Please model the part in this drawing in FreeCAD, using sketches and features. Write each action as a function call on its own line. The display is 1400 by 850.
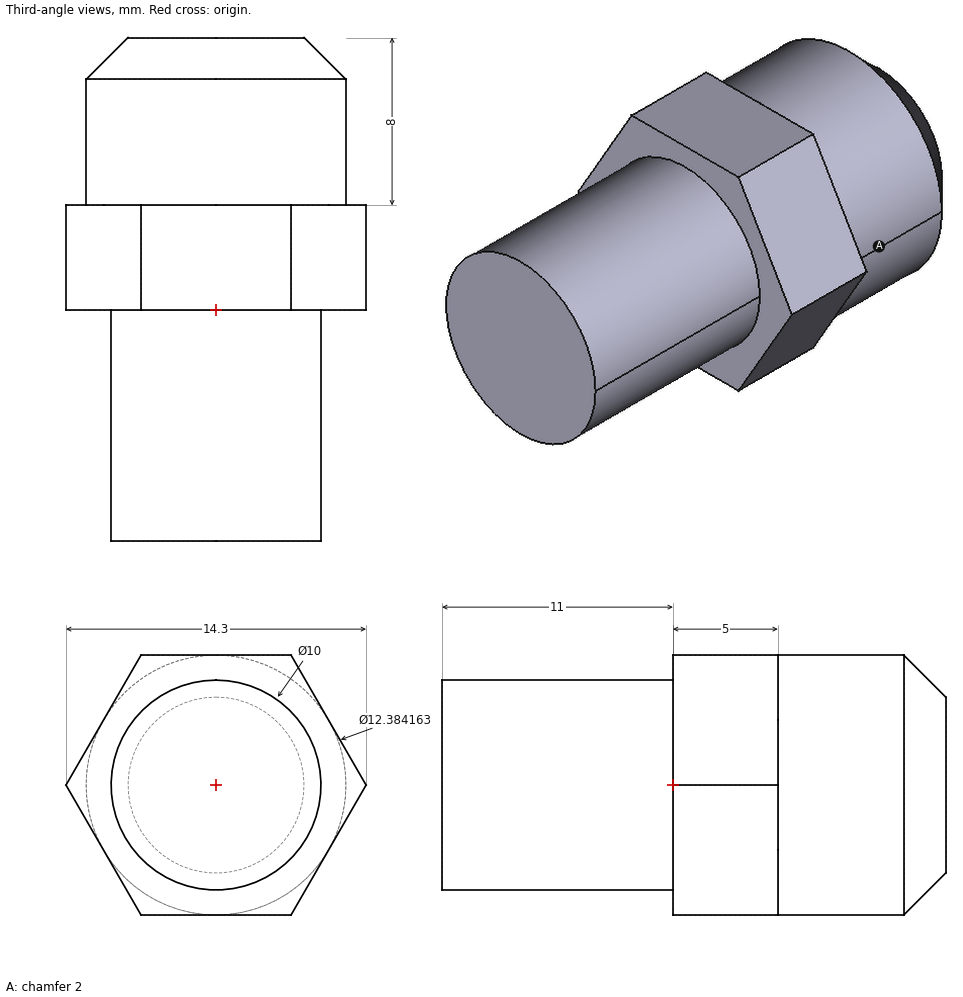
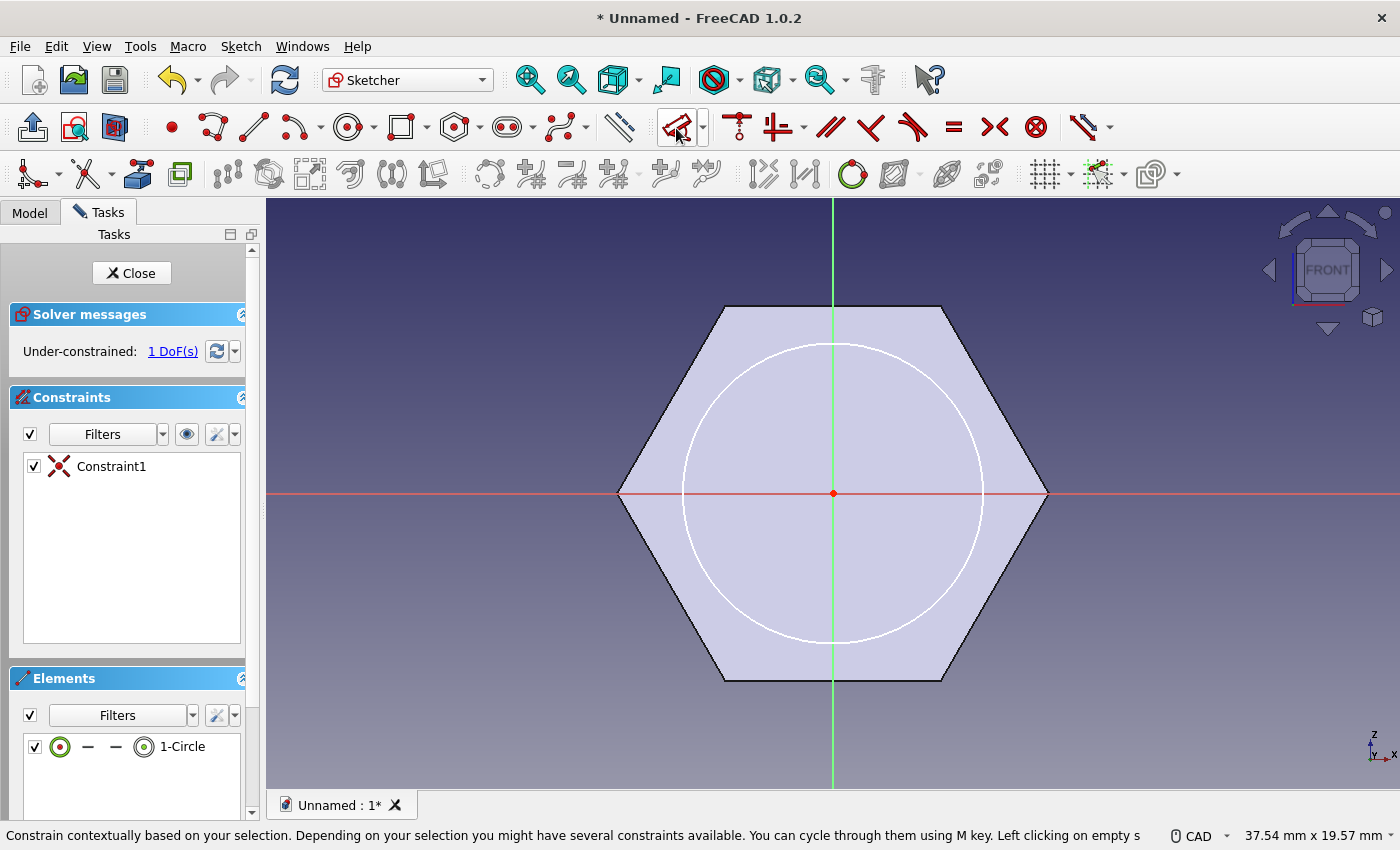
click(939, 387)
click(962, 364)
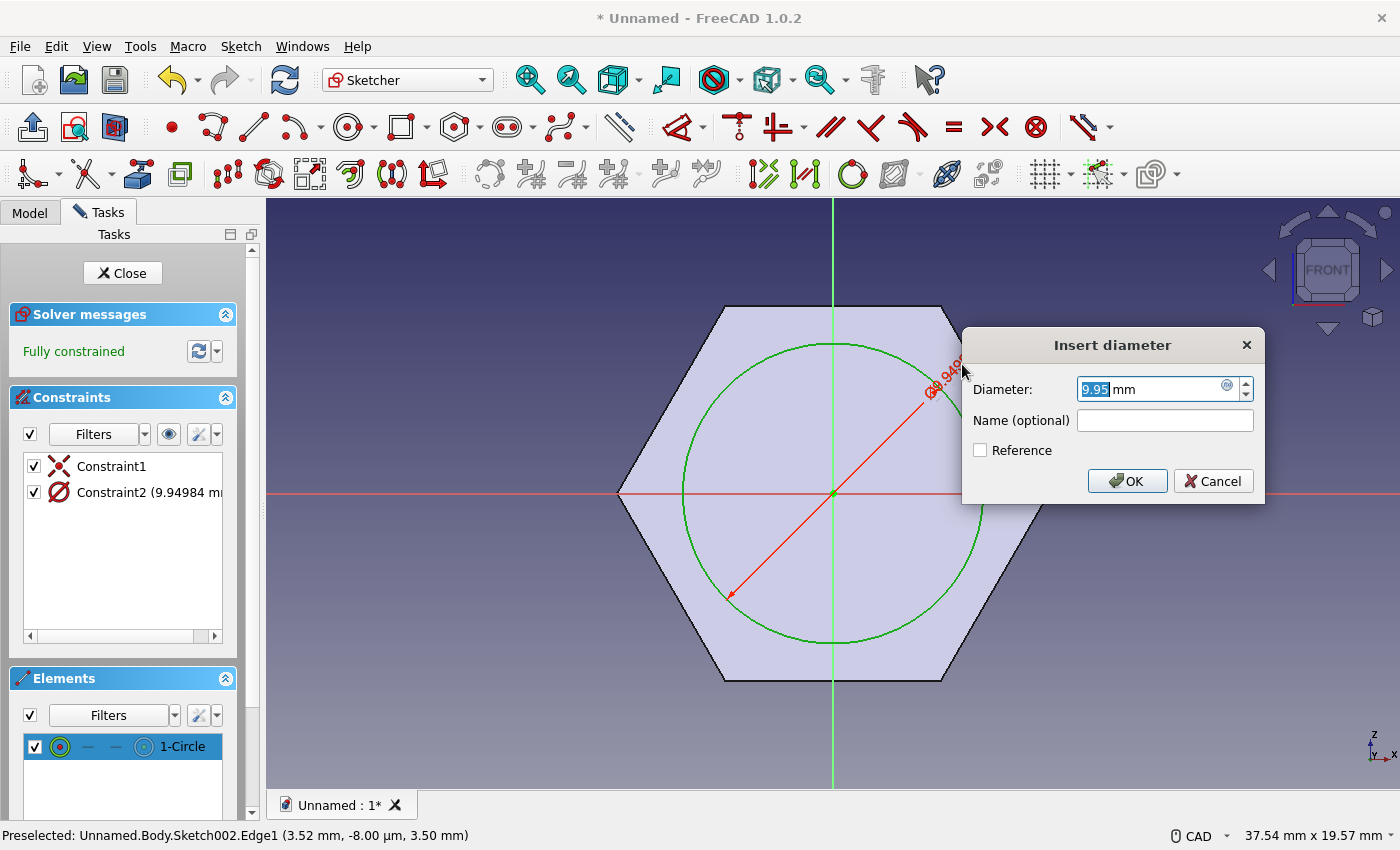
text(10)
key(Return)
key(Escape)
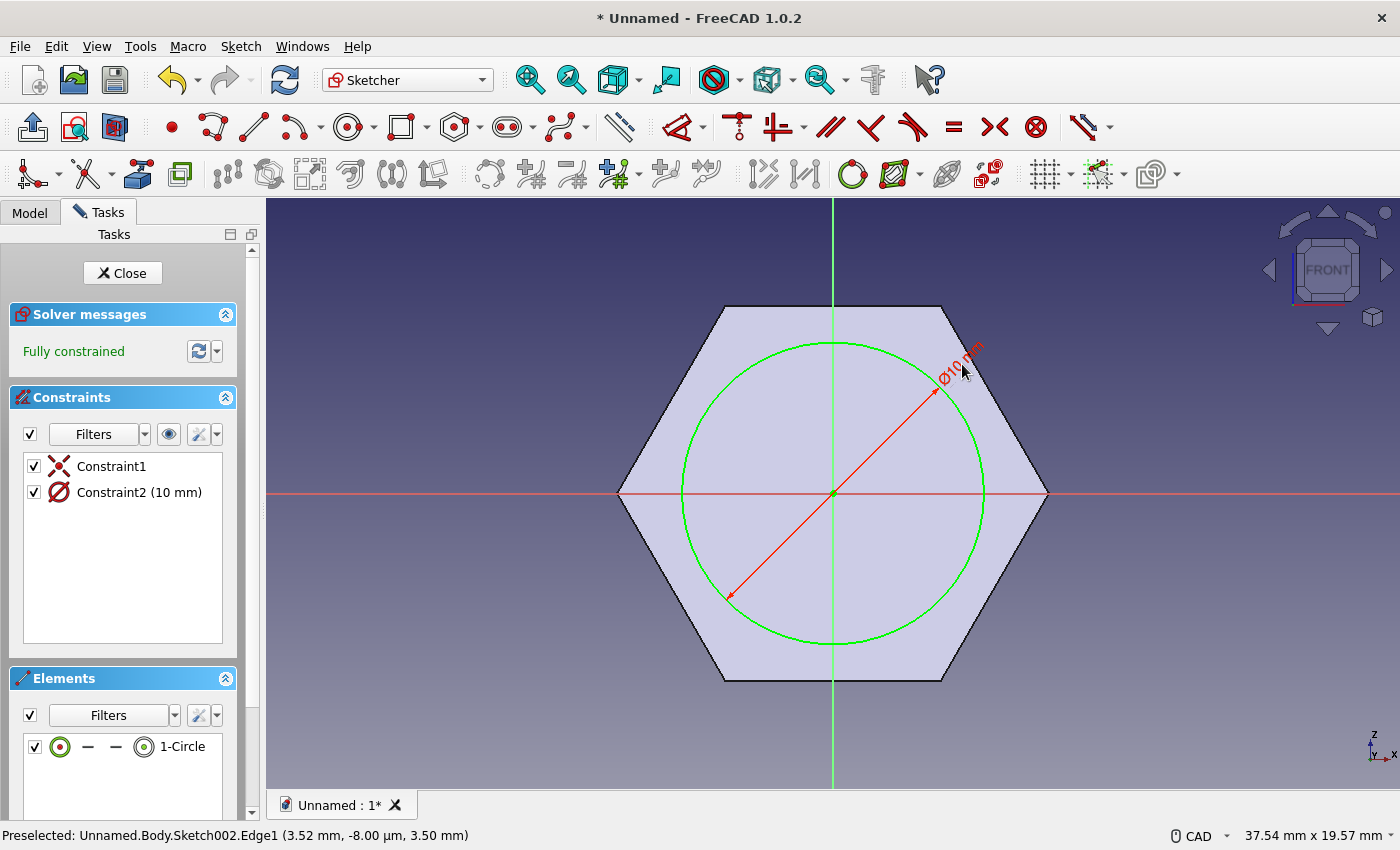
click(123, 273)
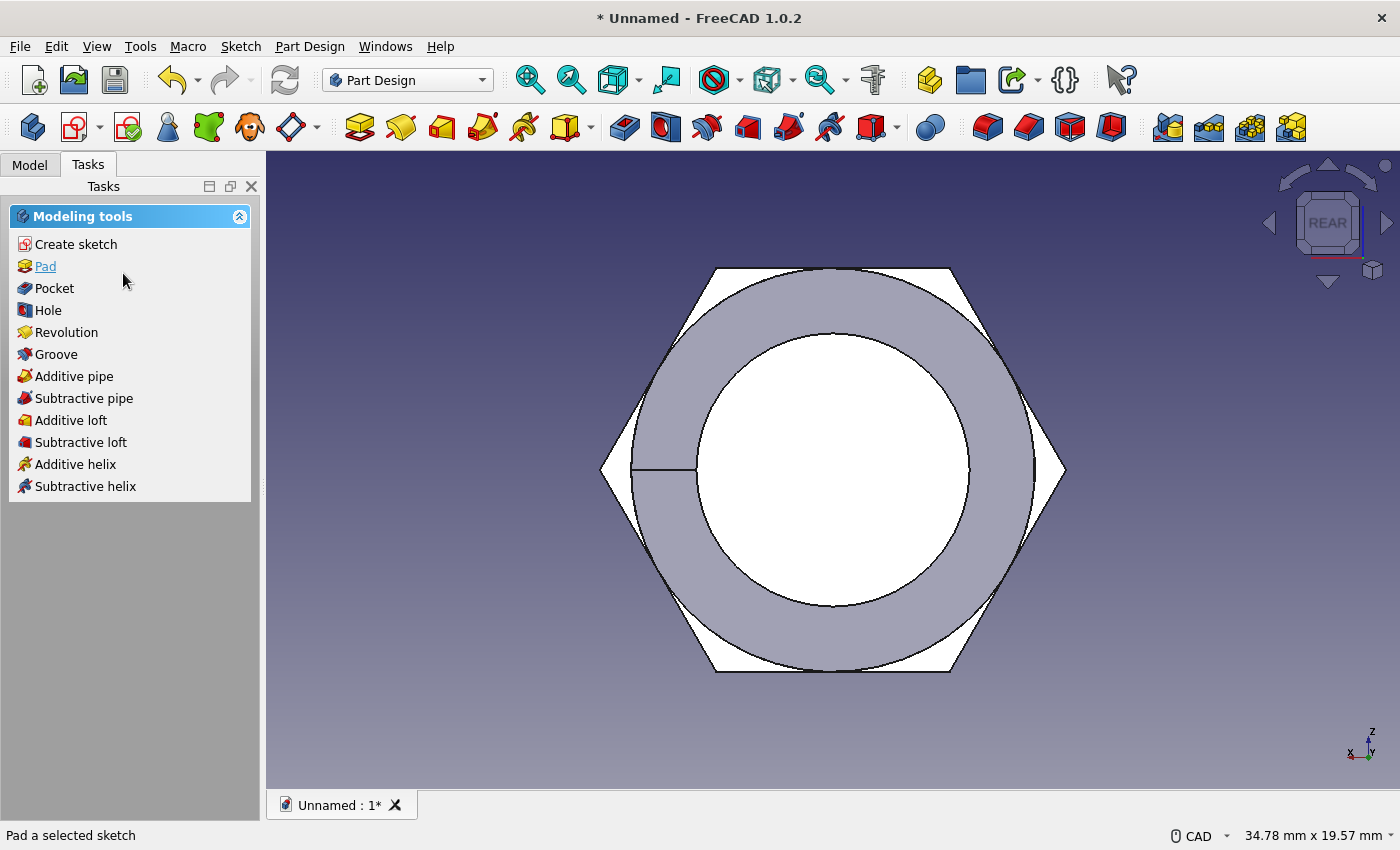
click(360, 128)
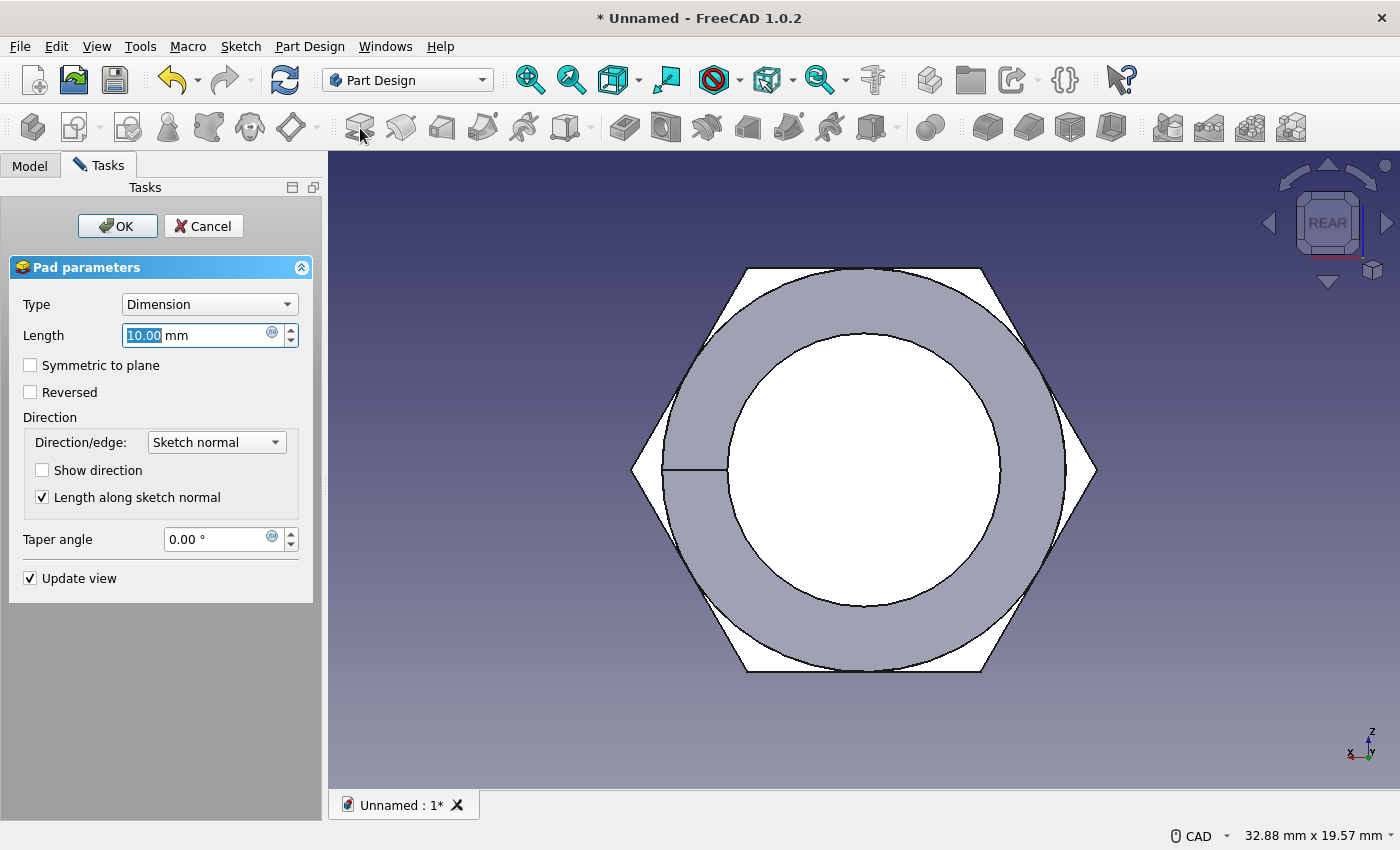
text(11)
key(Tab)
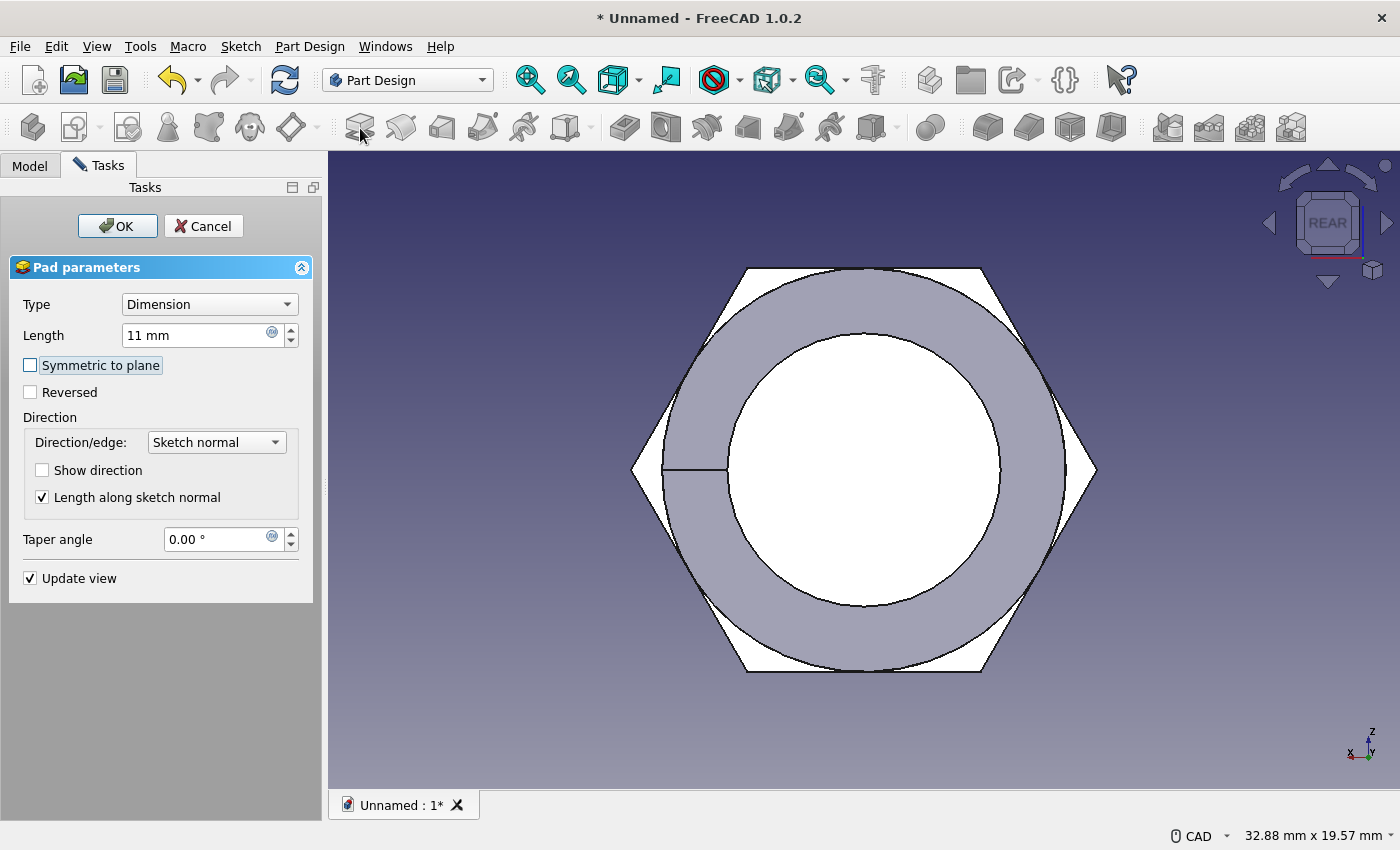
click(118, 226)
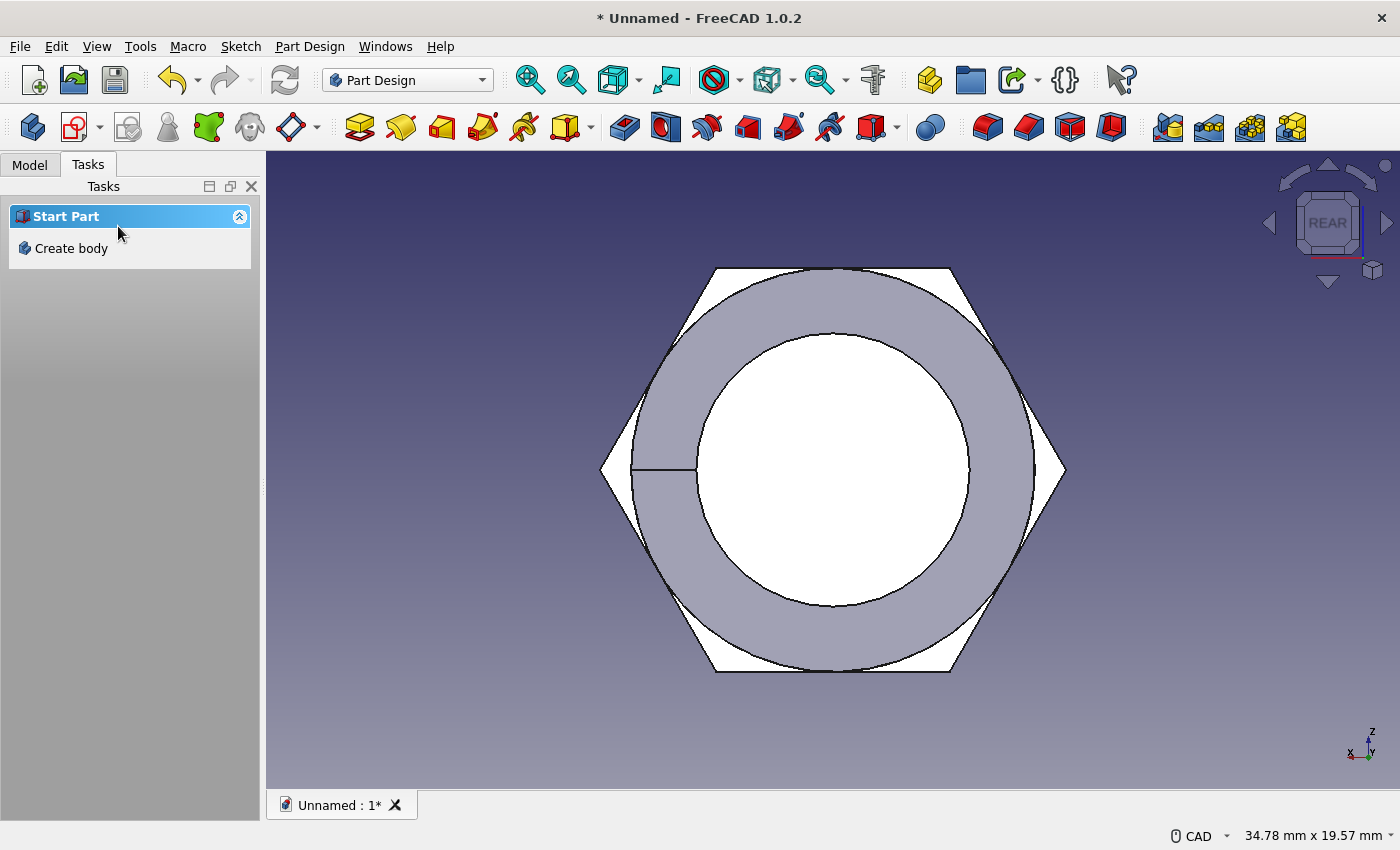
key(0)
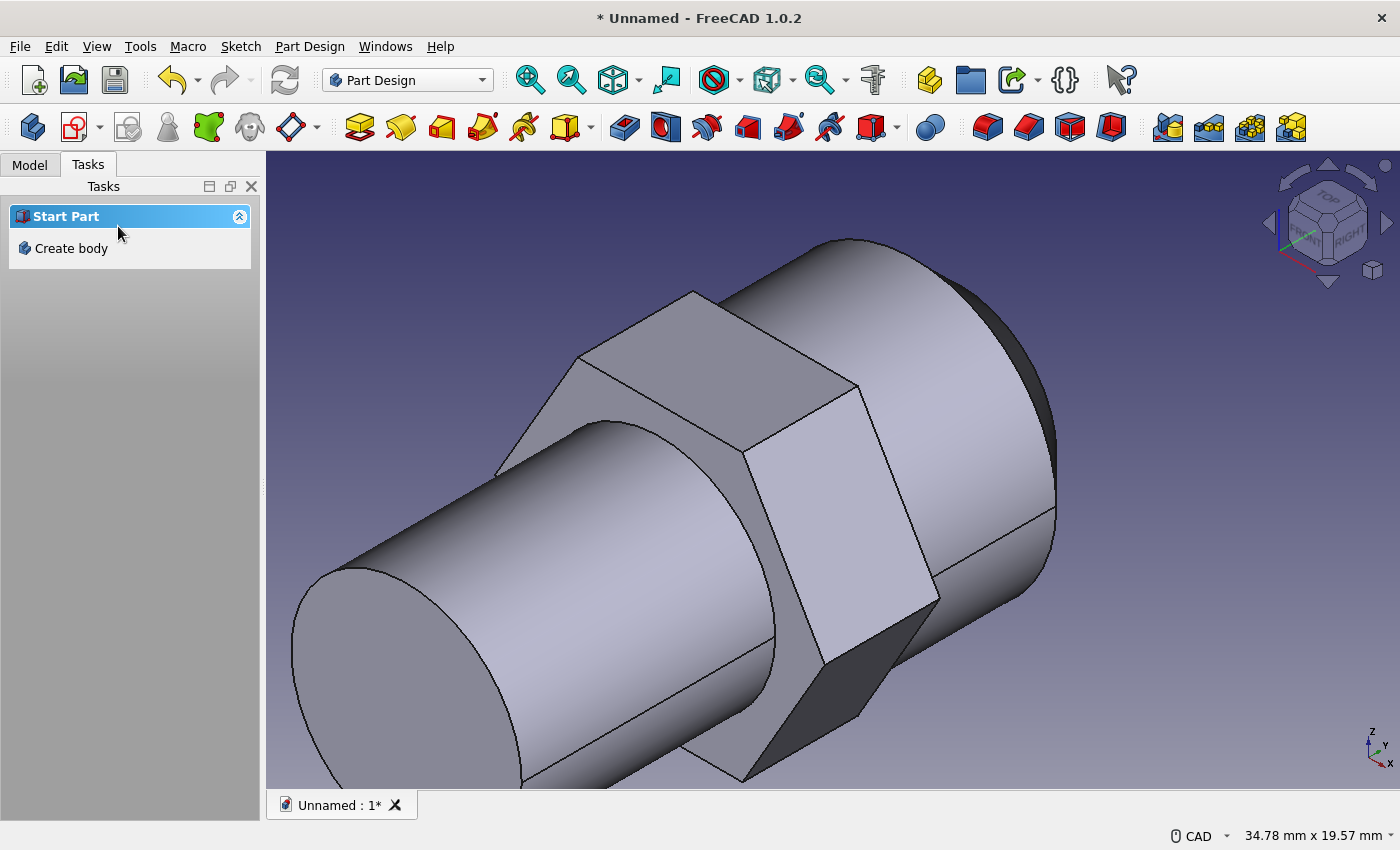
click(531, 80)